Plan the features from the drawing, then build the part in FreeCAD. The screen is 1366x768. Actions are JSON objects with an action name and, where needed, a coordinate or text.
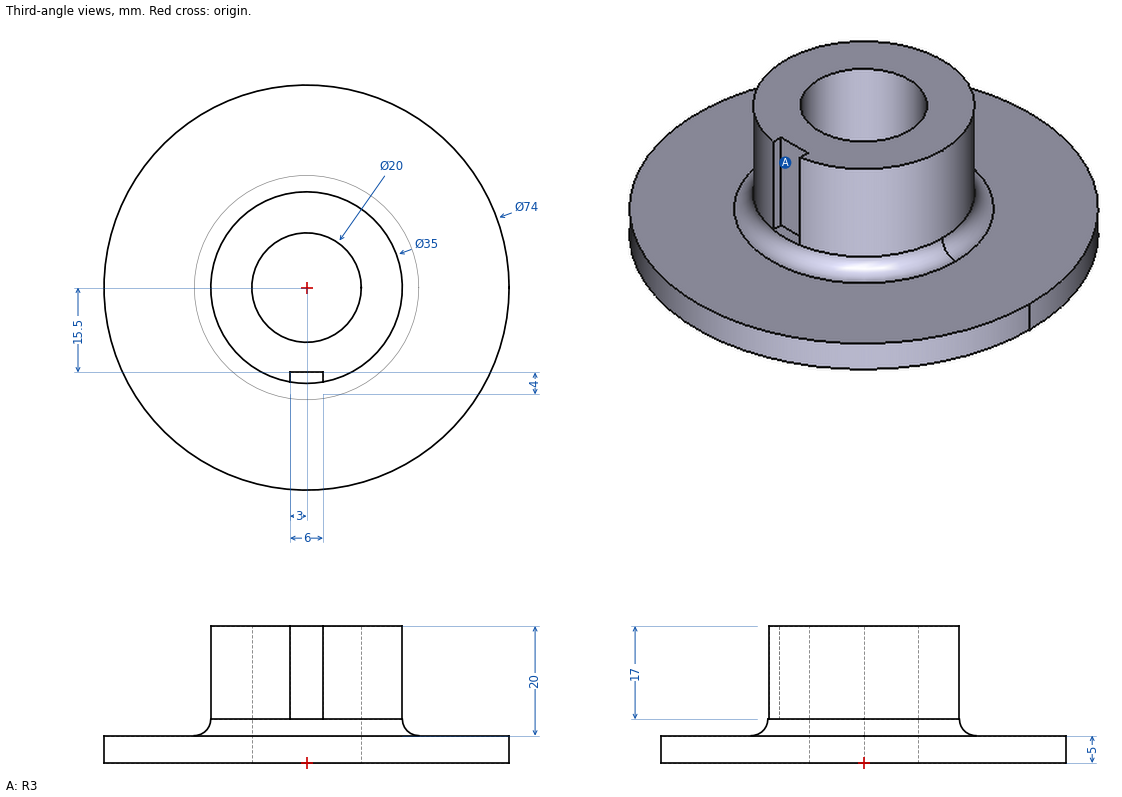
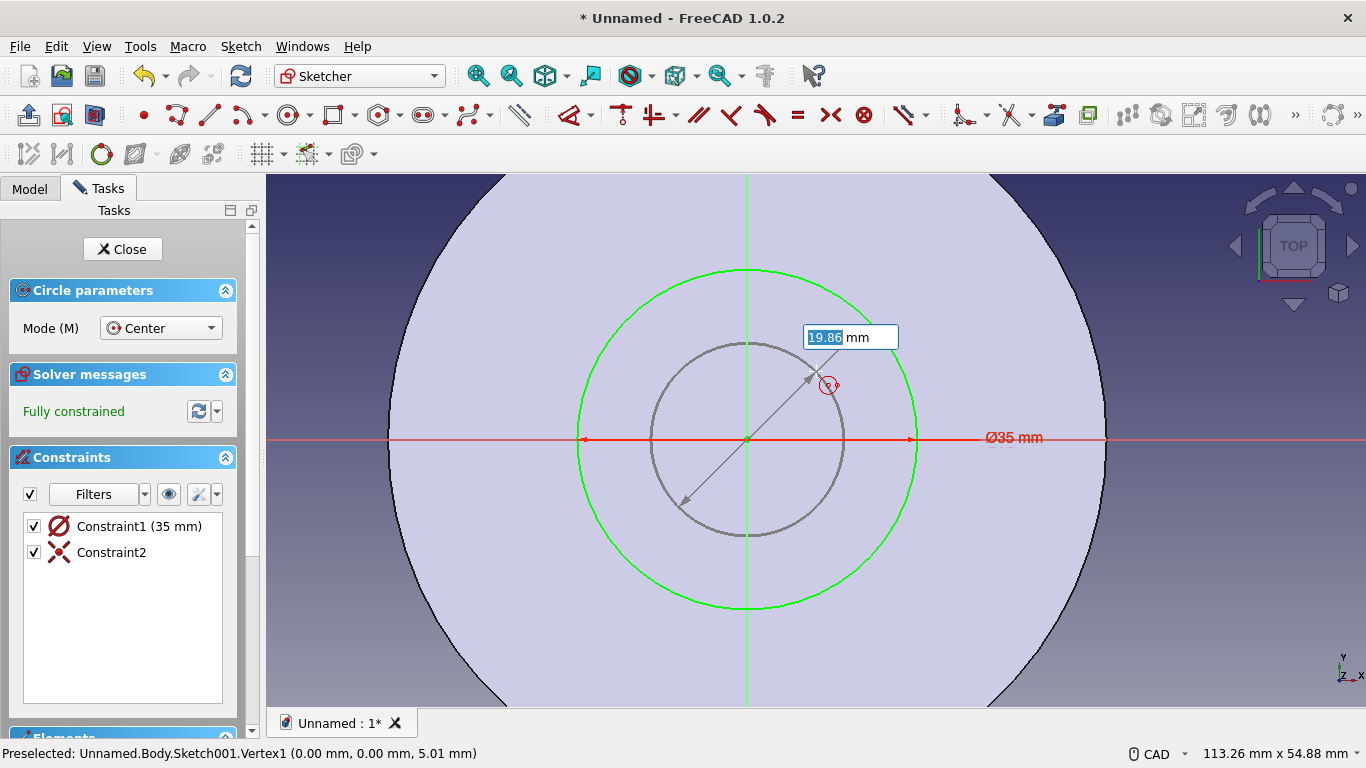
{"action": "type", "text": "20"}
{"action": "key", "text": "Return"}
{"action": "key", "text": "Escape"}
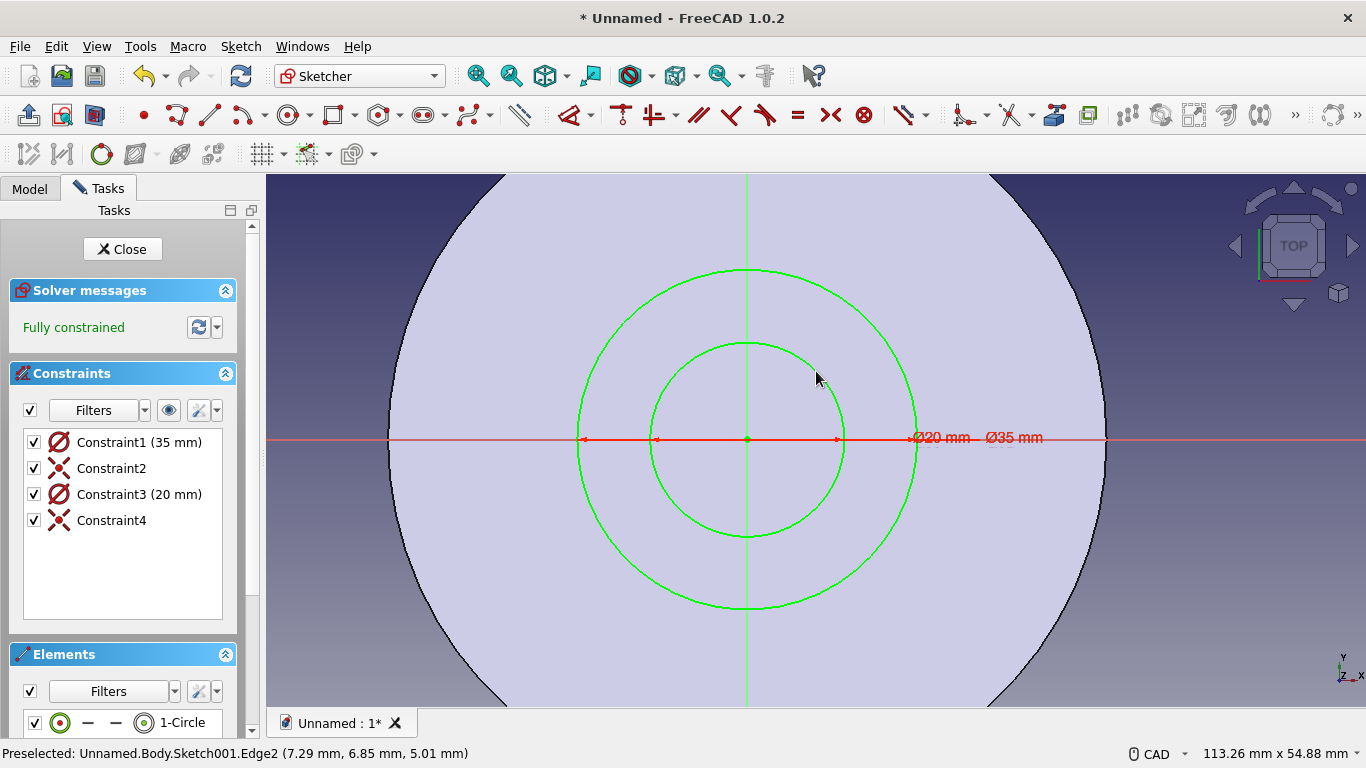
{"action": "left_click", "coordinate": [123, 249]}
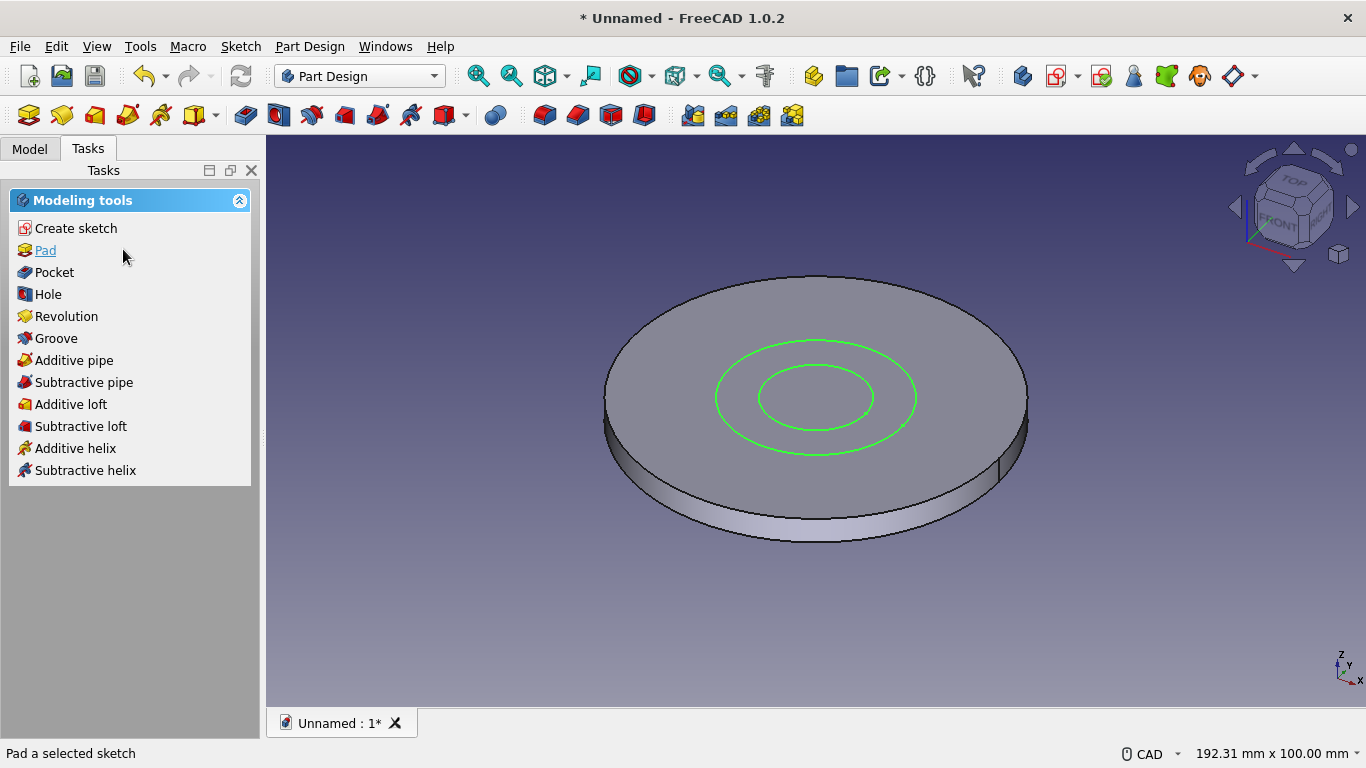
{"action": "left_click", "coordinate": [29, 116]}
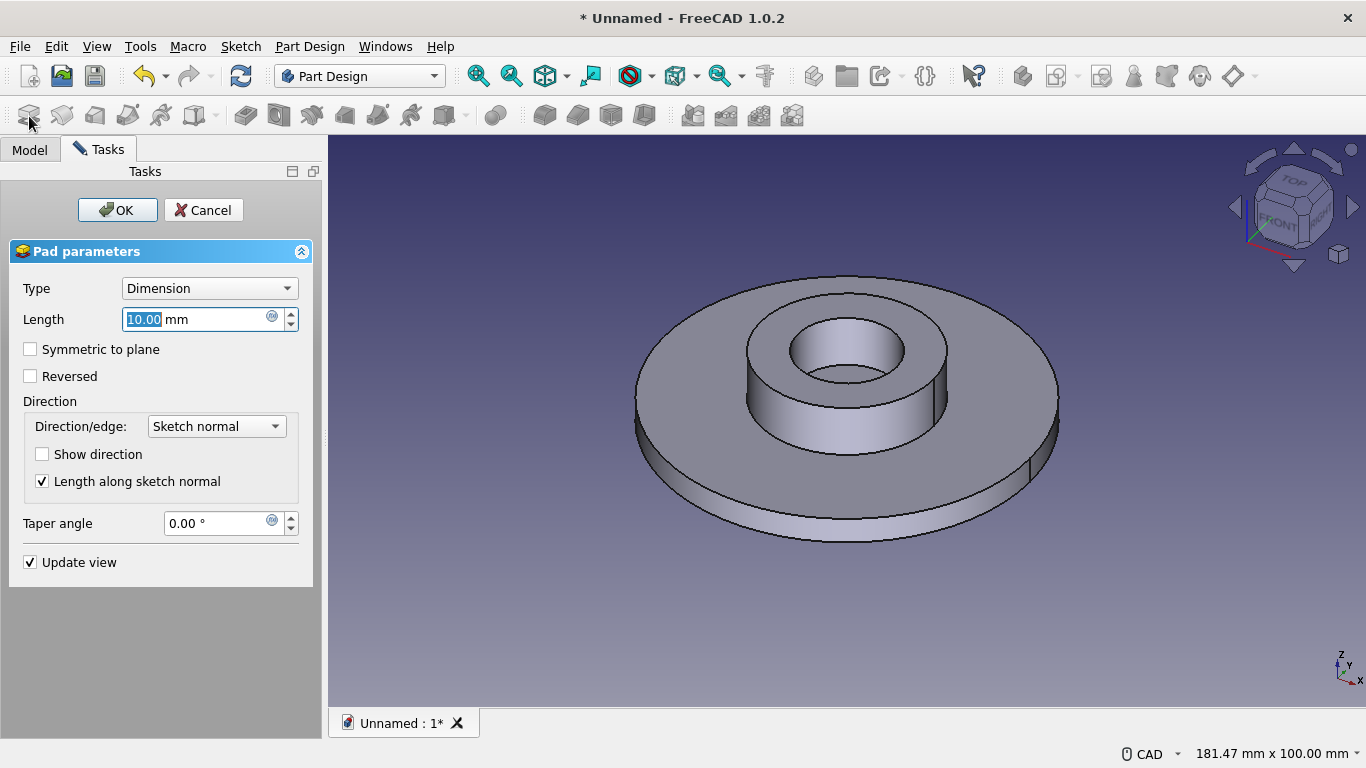
{"action": "type", "text": "20"}
{"action": "key", "text": "Tab"}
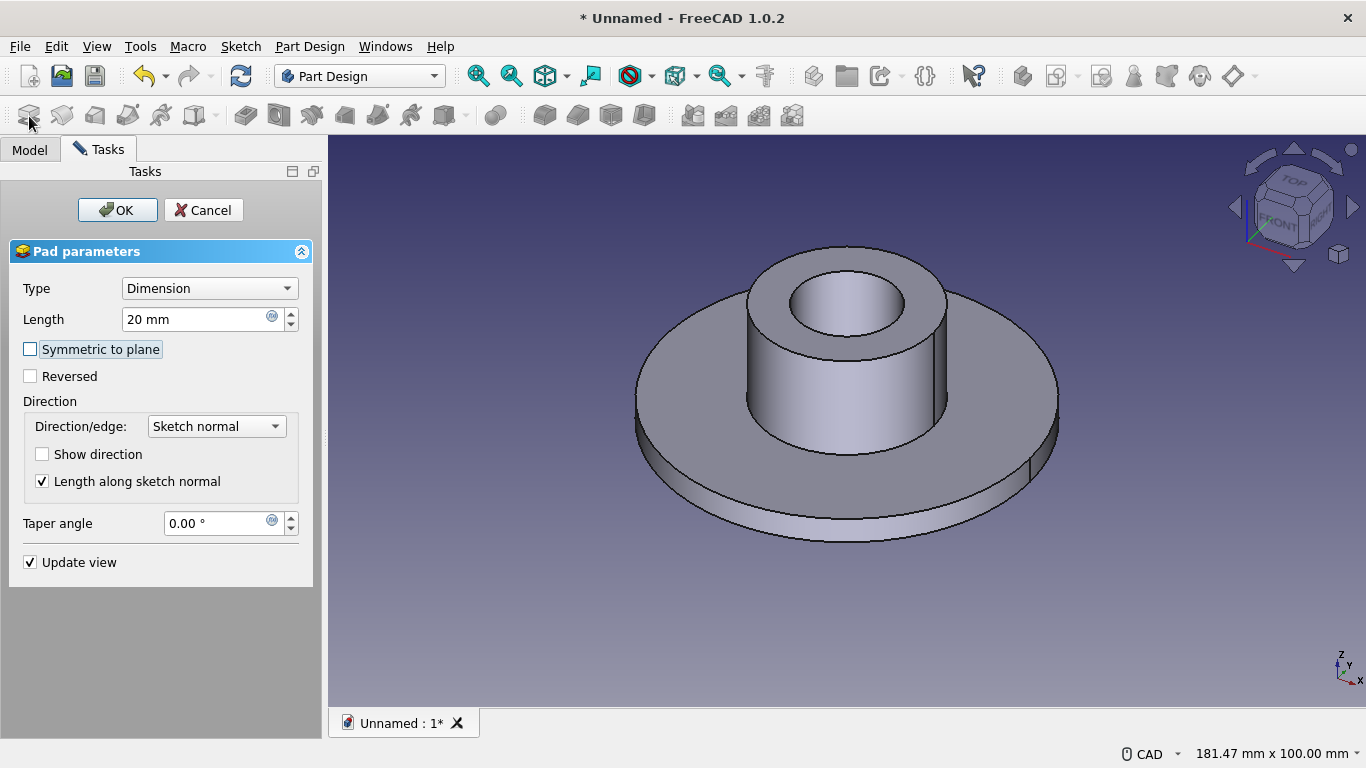
{"action": "left_click", "coordinate": [118, 210]}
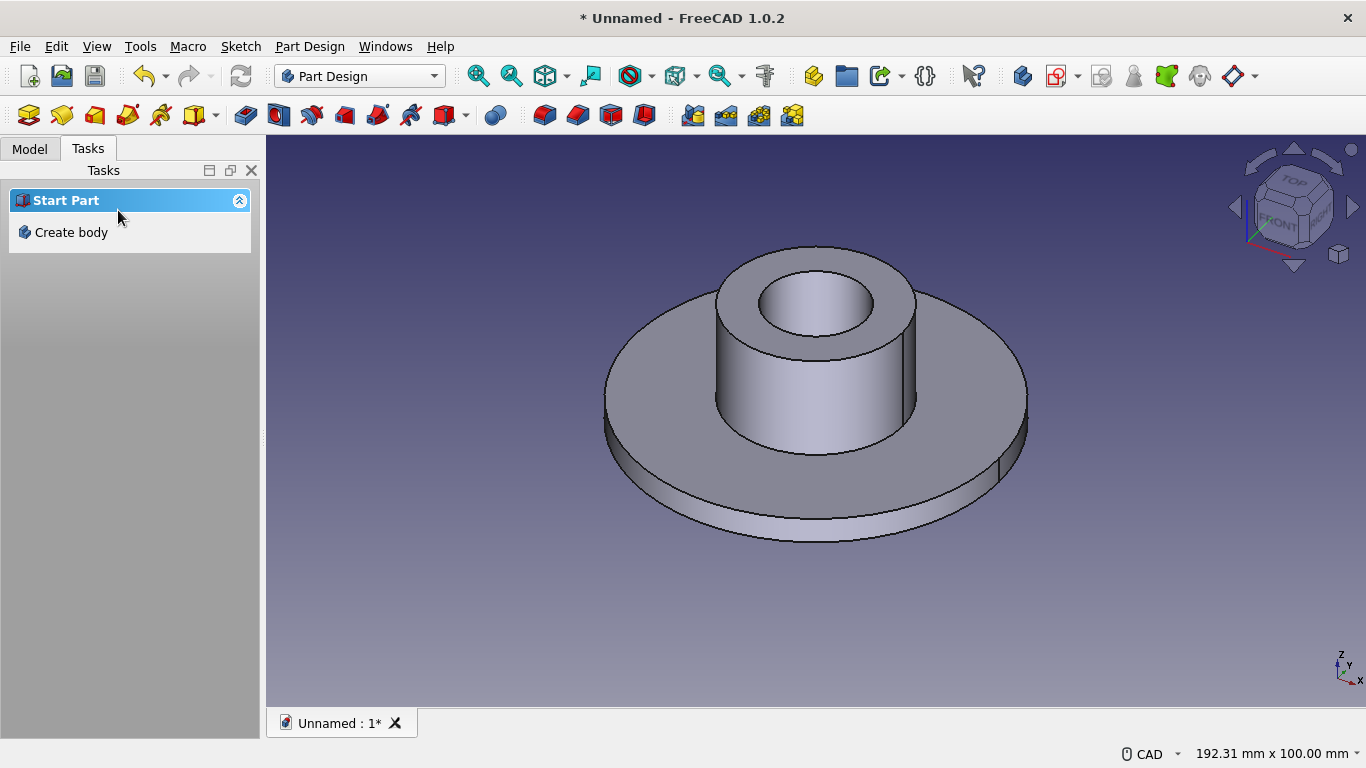
{"action": "left_click", "coordinate": [738, 315]}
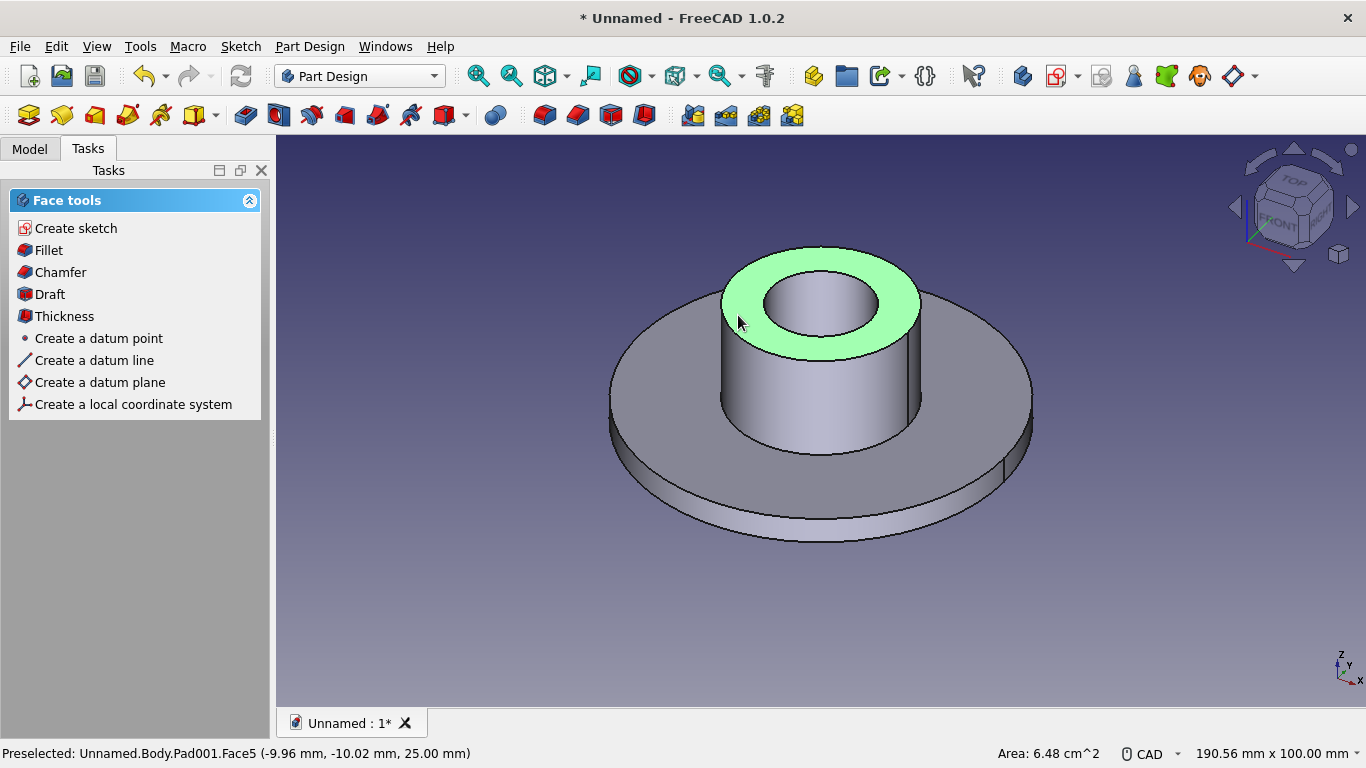
{"action": "left_click", "coordinate": [1056, 76]}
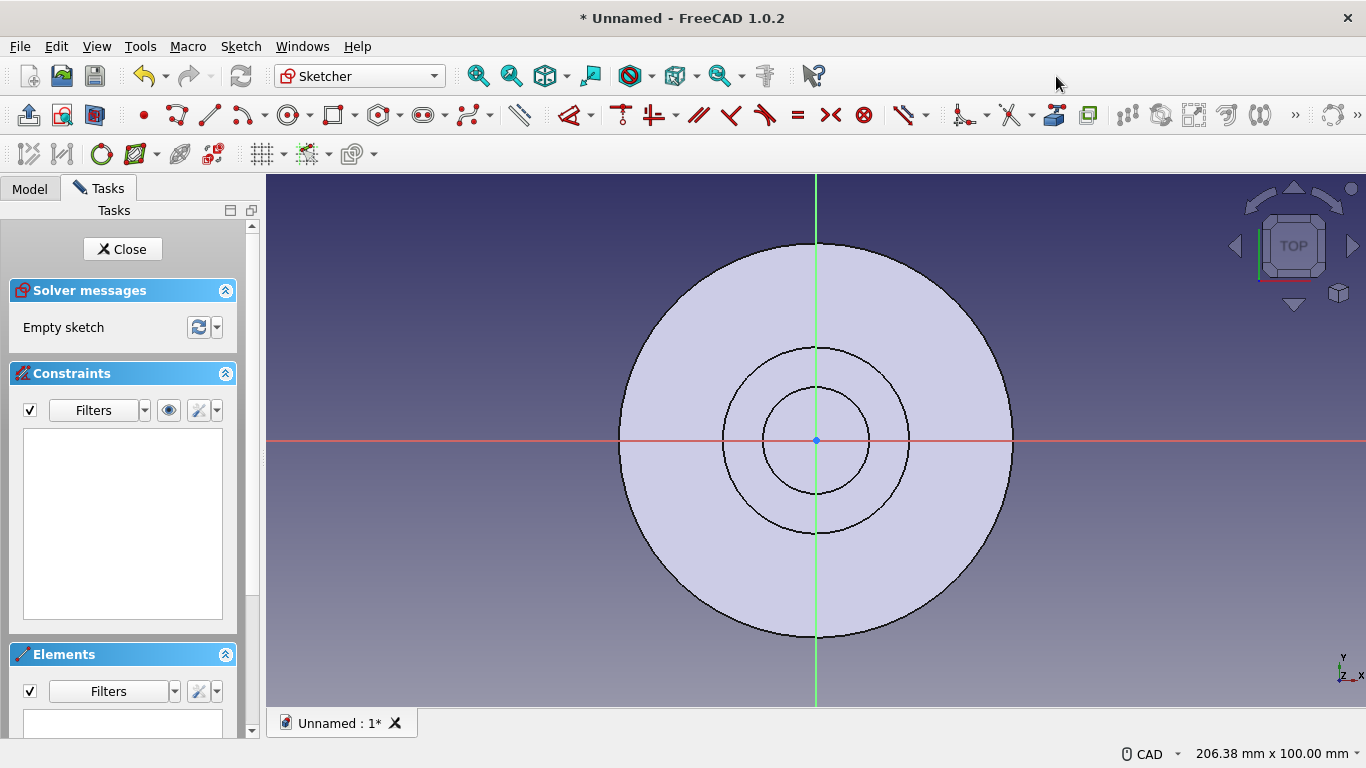
{"action": "scroll", "coordinate": [846, 440], "scroll_direction": "up", "scroll_amount": 6}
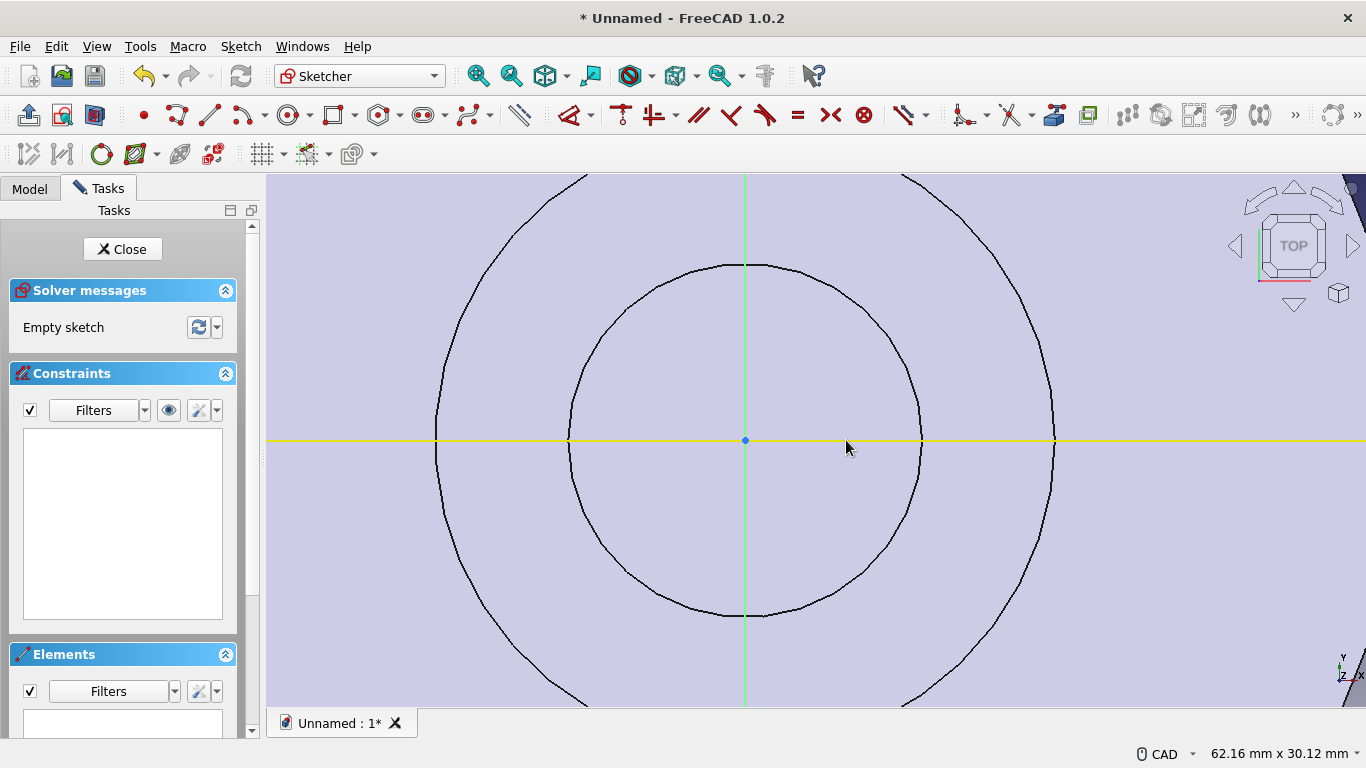
{"action": "left_click", "coordinate": [288, 116]}